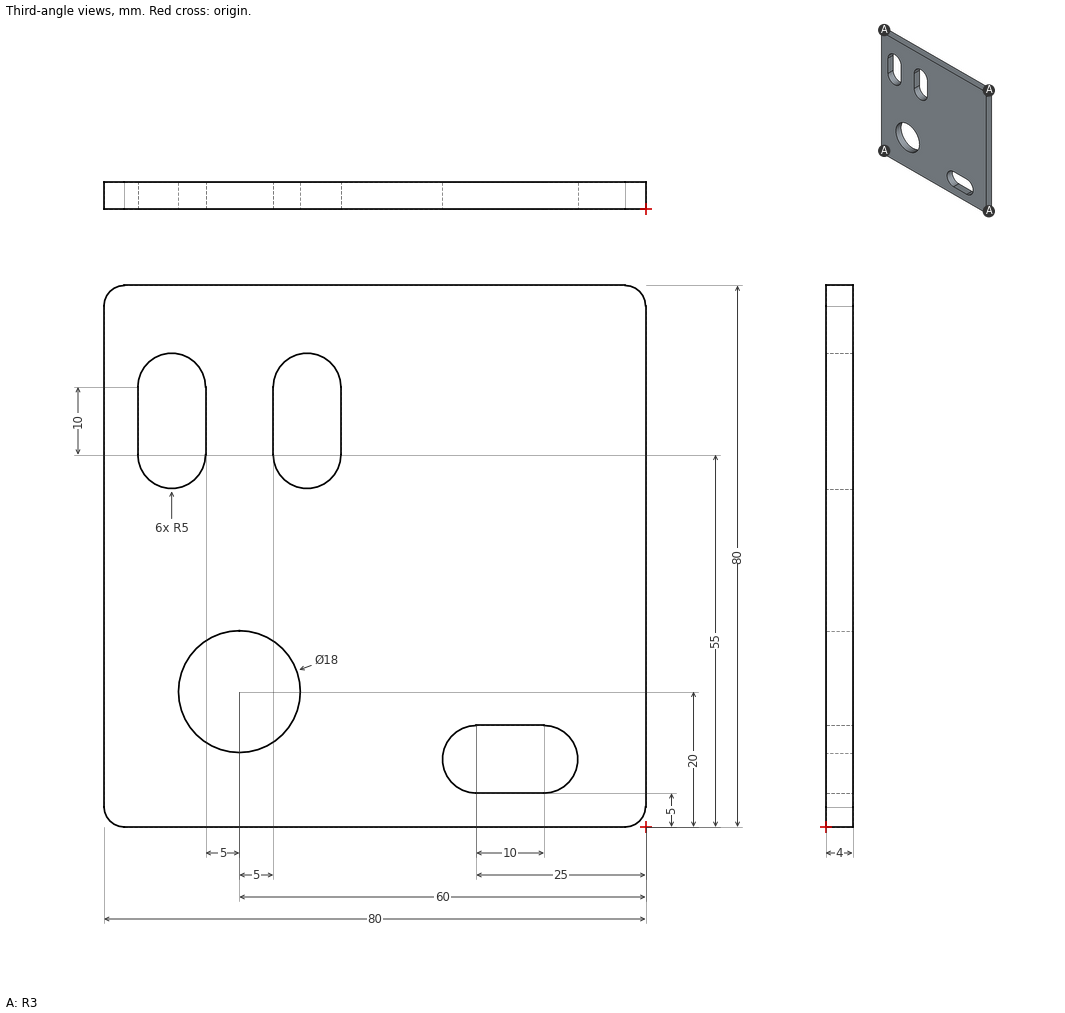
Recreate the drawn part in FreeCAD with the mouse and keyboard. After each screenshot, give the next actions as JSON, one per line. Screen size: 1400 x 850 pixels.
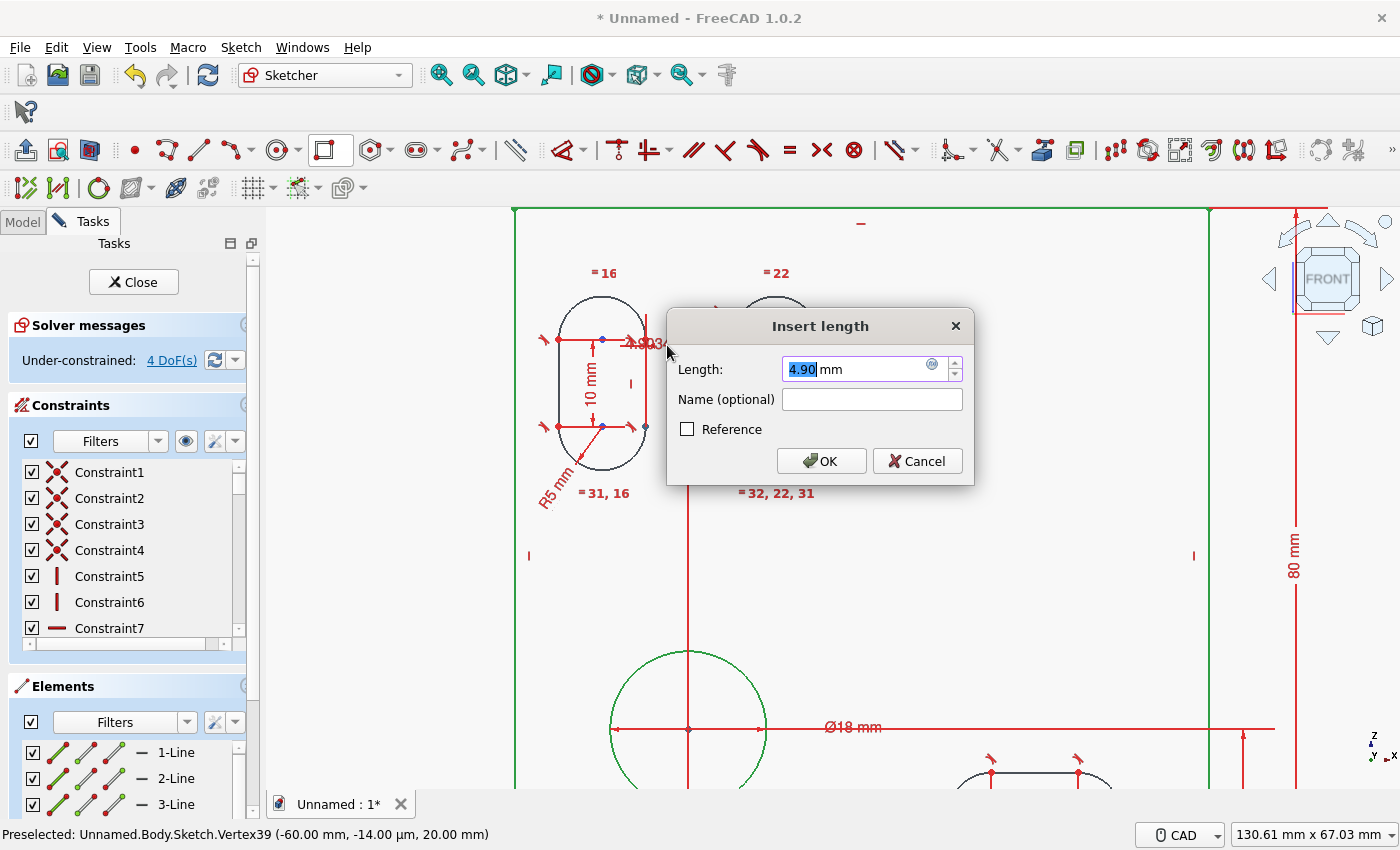
{"action": "type", "text": "5"}
{"action": "key", "text": "Return"}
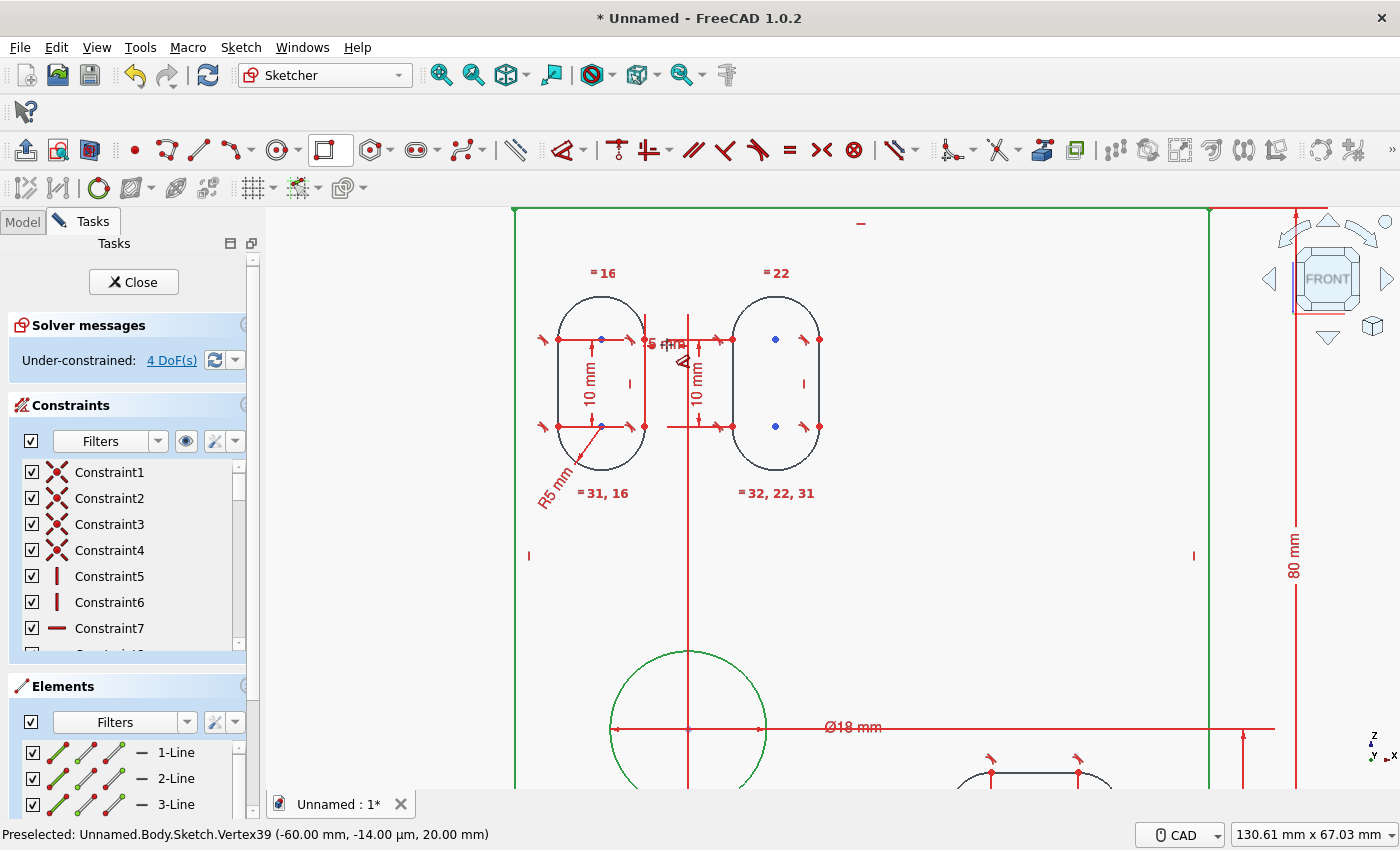
{"action": "left_click", "coordinate": [733, 427]}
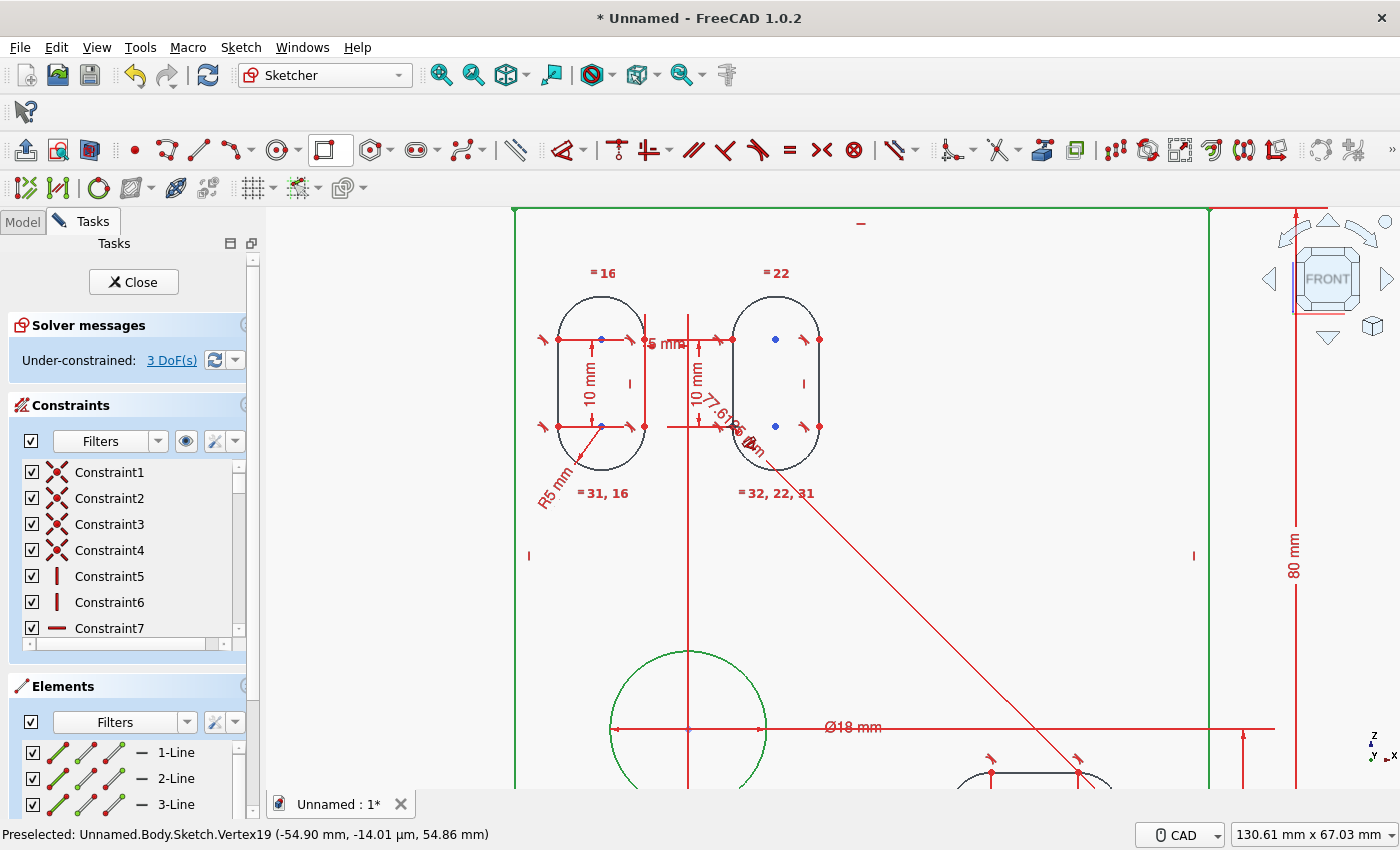
{"action": "left_click", "coordinate": [688, 729]}
{"action": "left_click", "coordinate": [710, 321]}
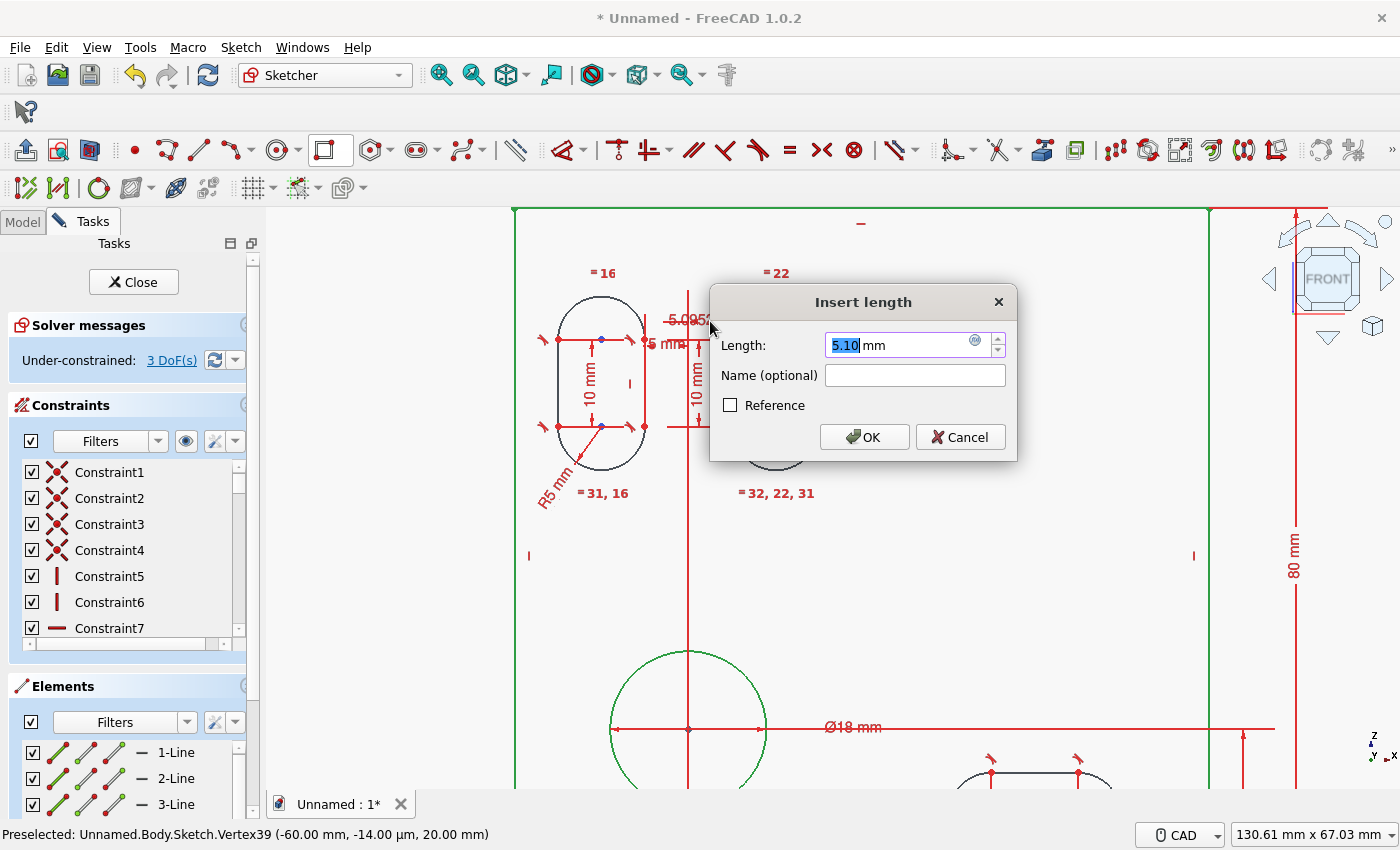
{"action": "type", "text": "5"}
{"action": "key", "text": "Return"}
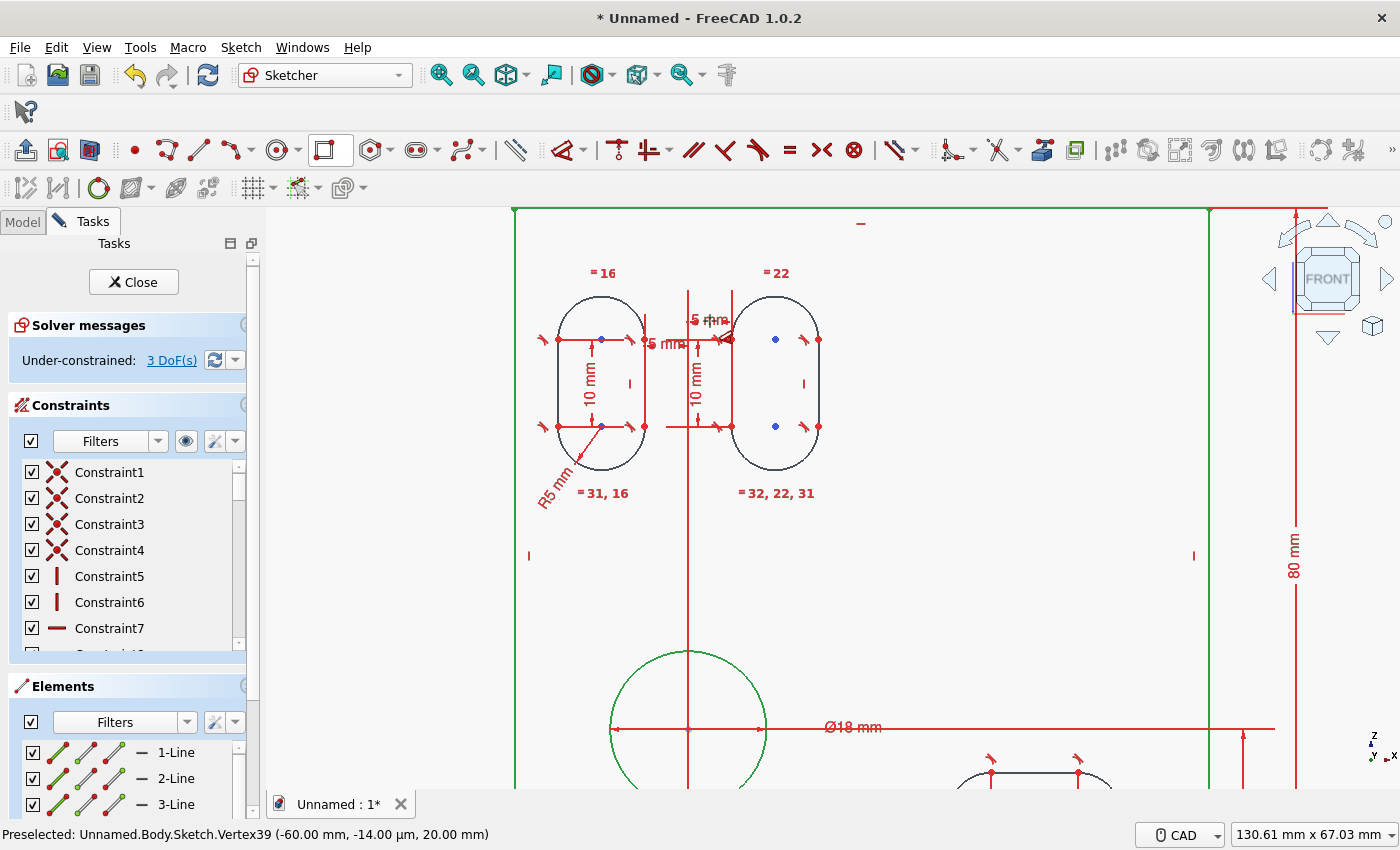
{"action": "left_click", "coordinate": [558, 427]}
{"action": "left_click", "coordinate": [500, 594]}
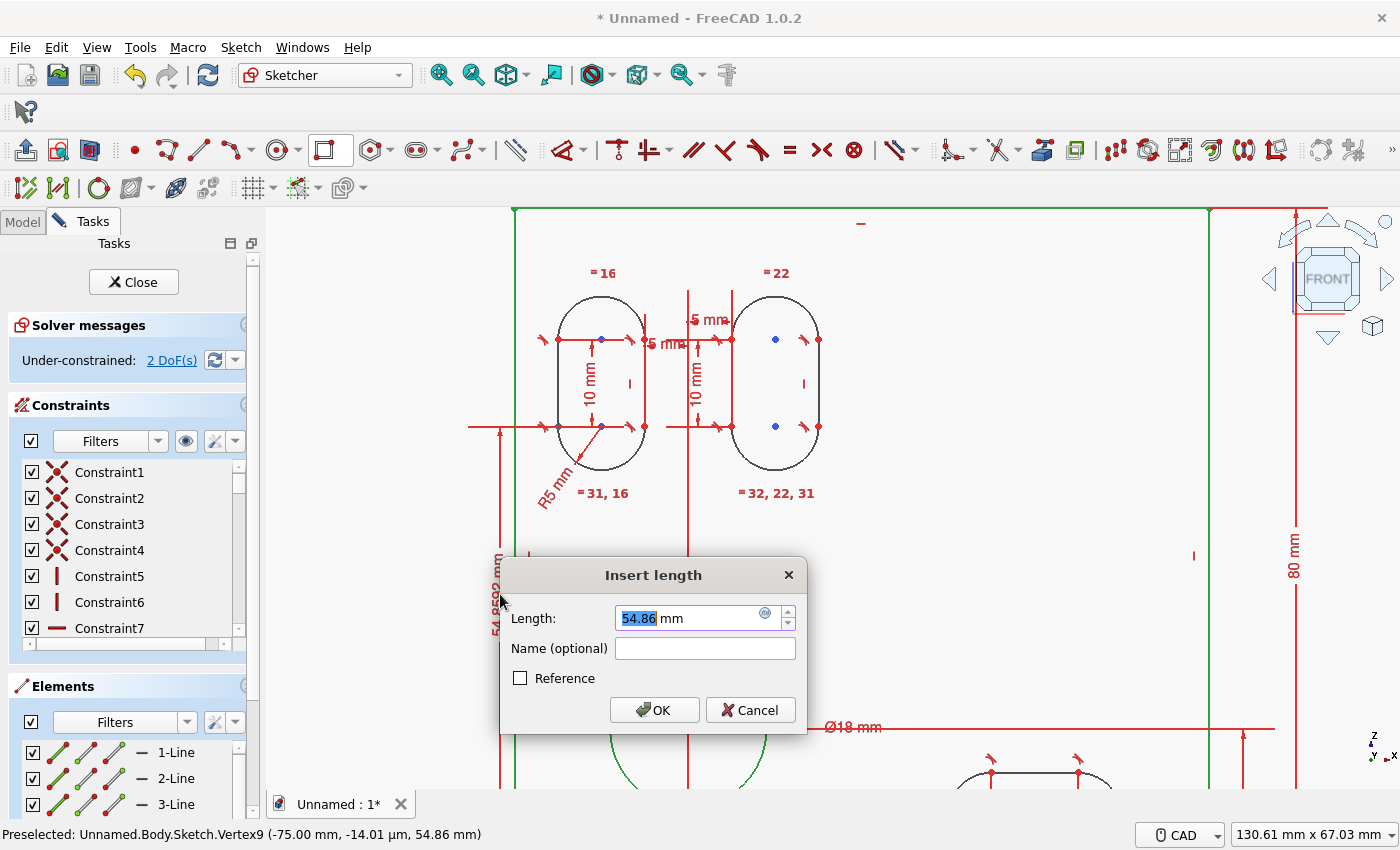
{"action": "type", "text": "55"}
{"action": "key", "text": "Return"}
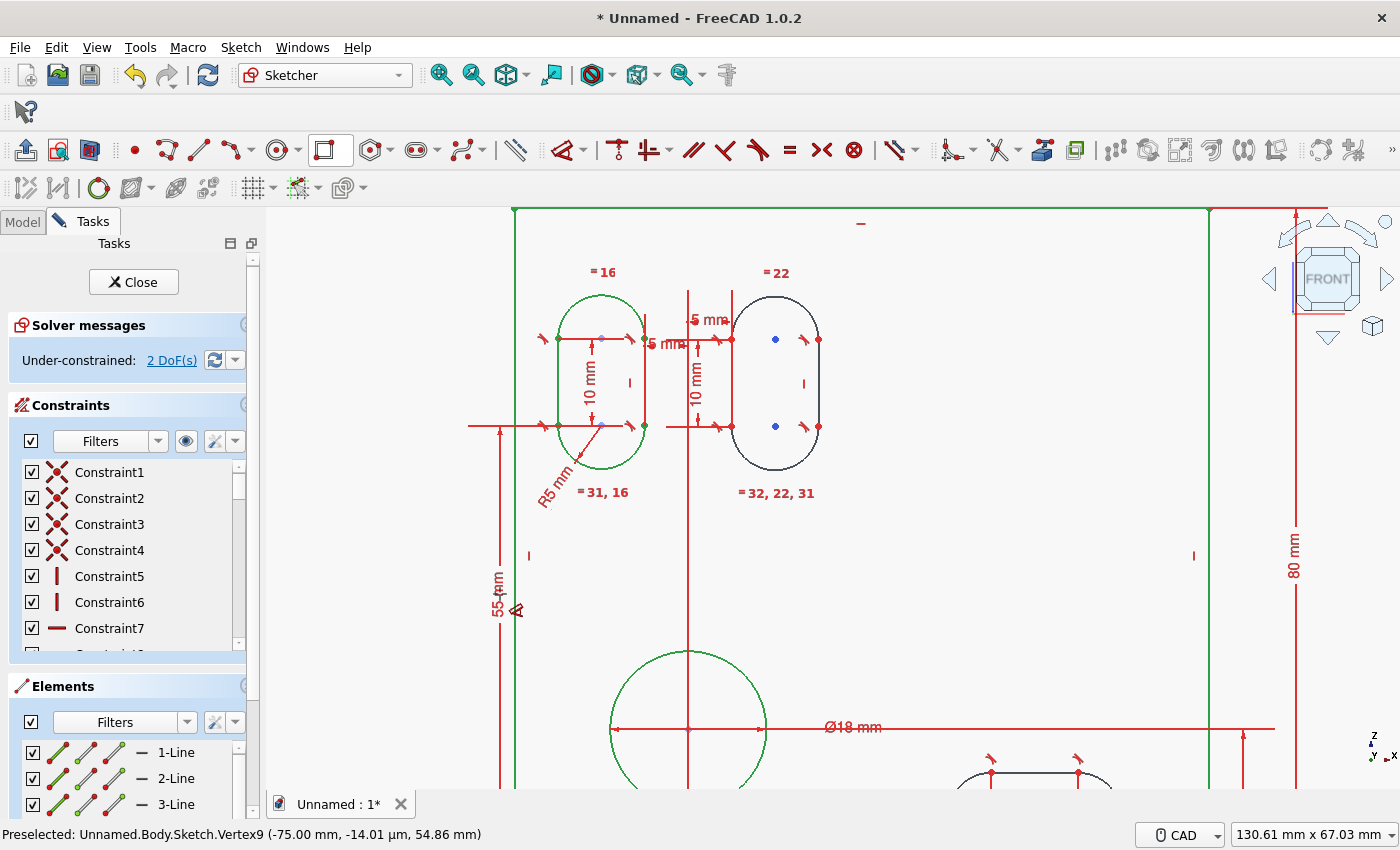
{"action": "left_click", "coordinate": [732, 427]}
{"action": "left_click", "coordinate": [698, 594]}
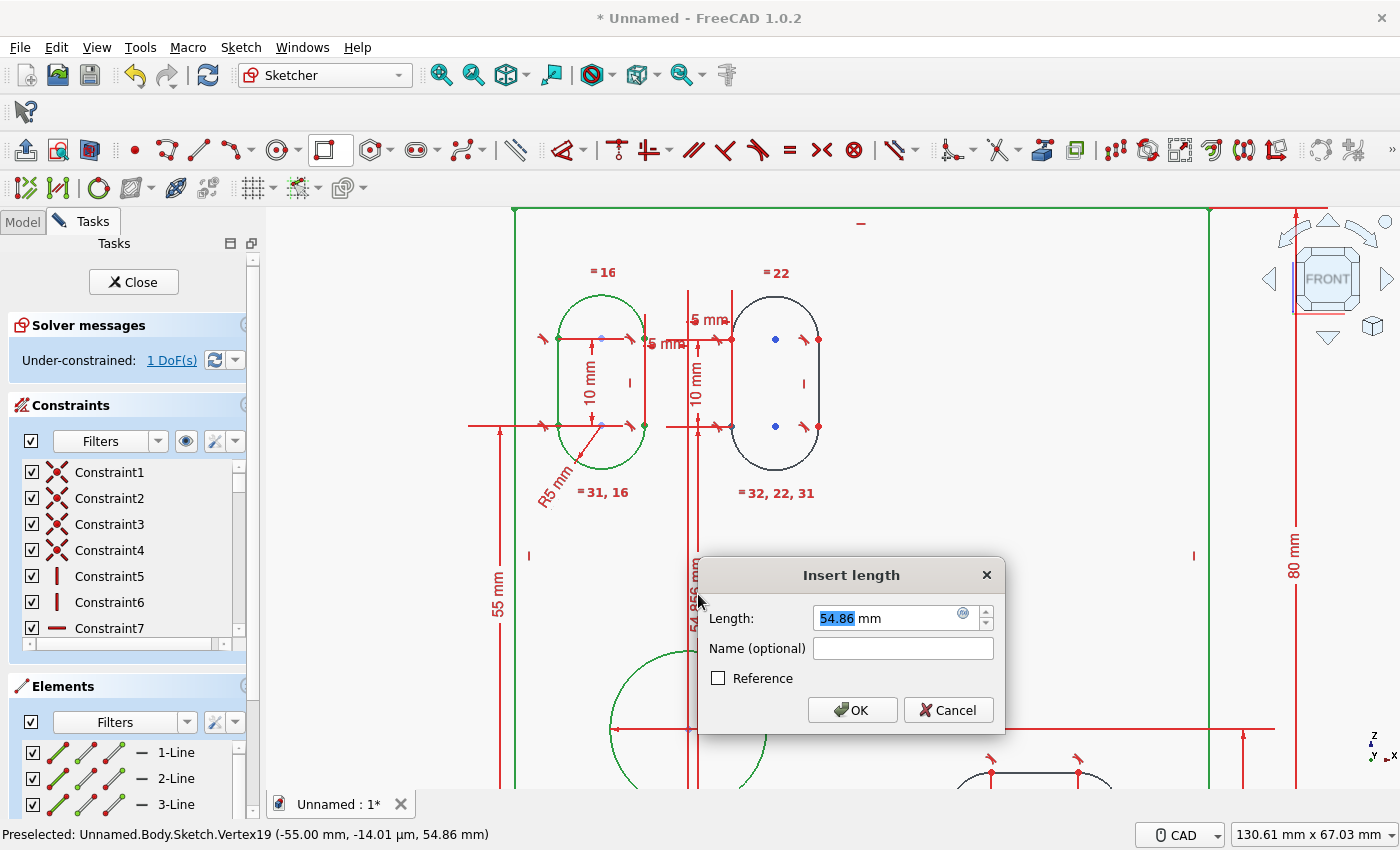
{"action": "type", "text": "55"}
{"action": "key", "text": "Return"}